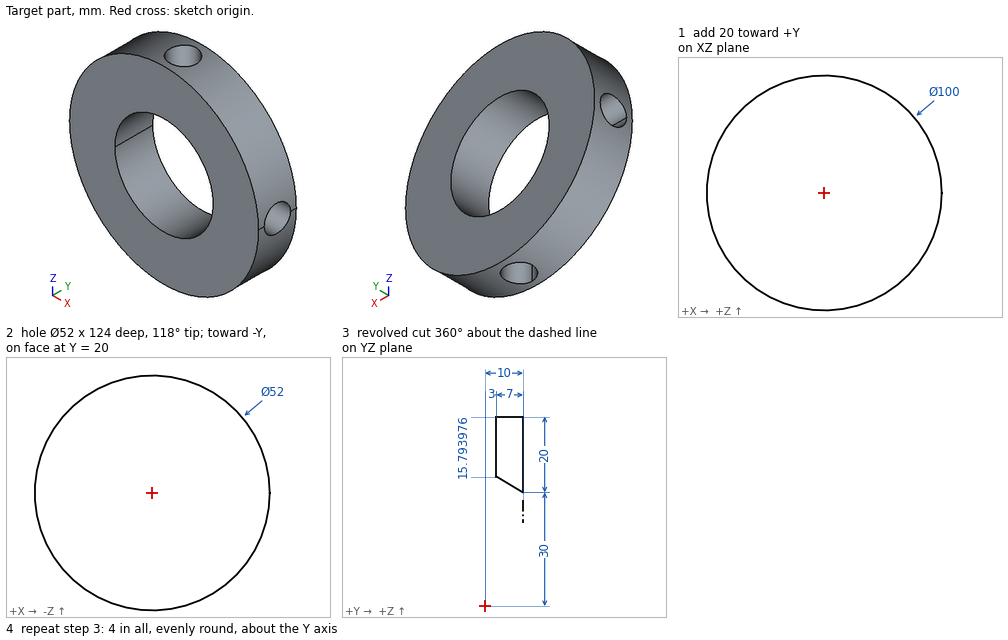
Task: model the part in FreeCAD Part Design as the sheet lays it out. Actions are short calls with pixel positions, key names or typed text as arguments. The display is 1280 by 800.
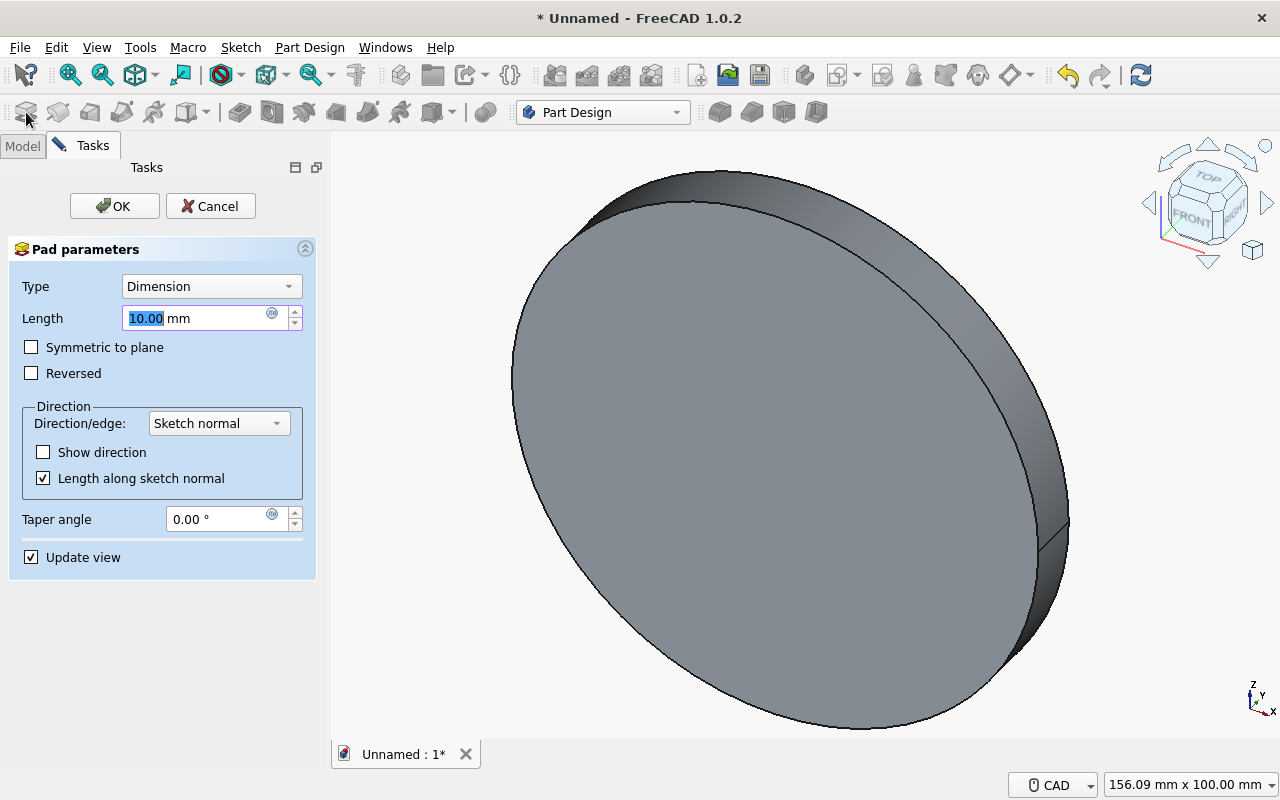
text(20)
key(Tab)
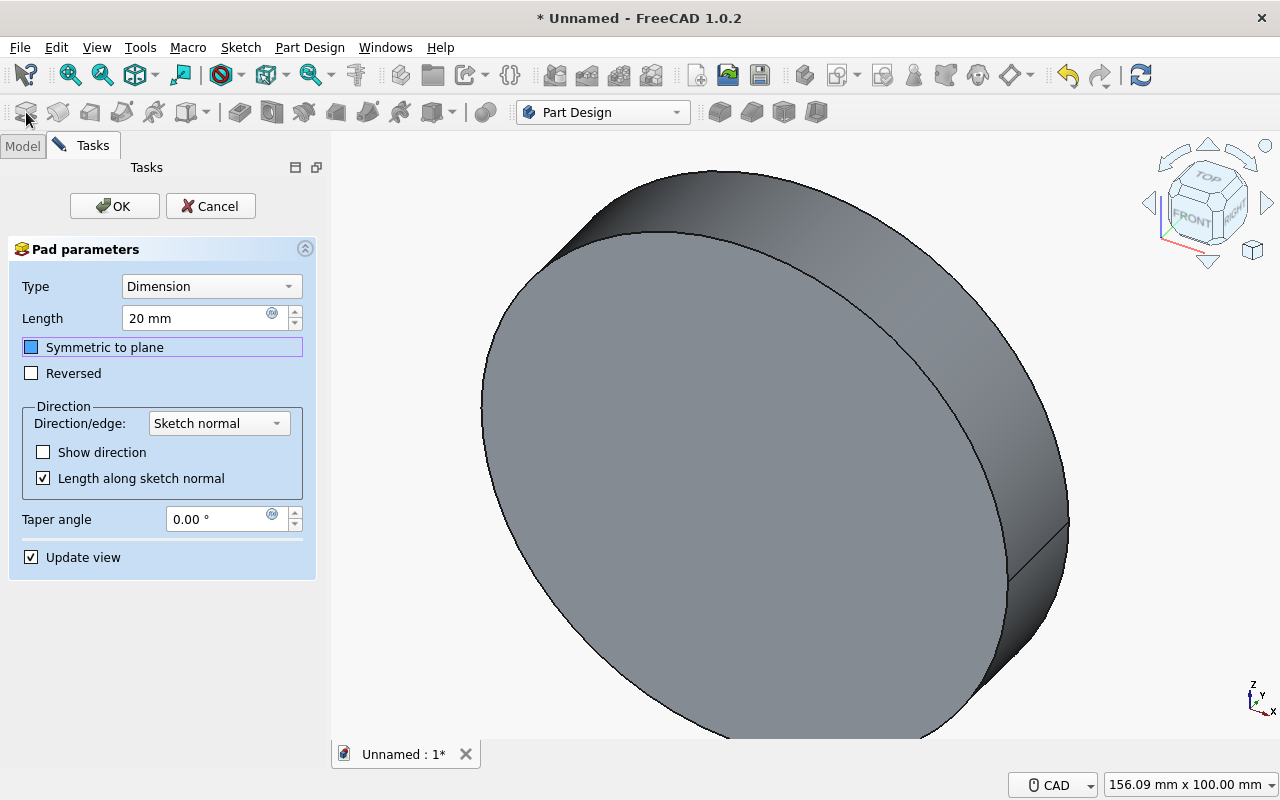
click(30, 373)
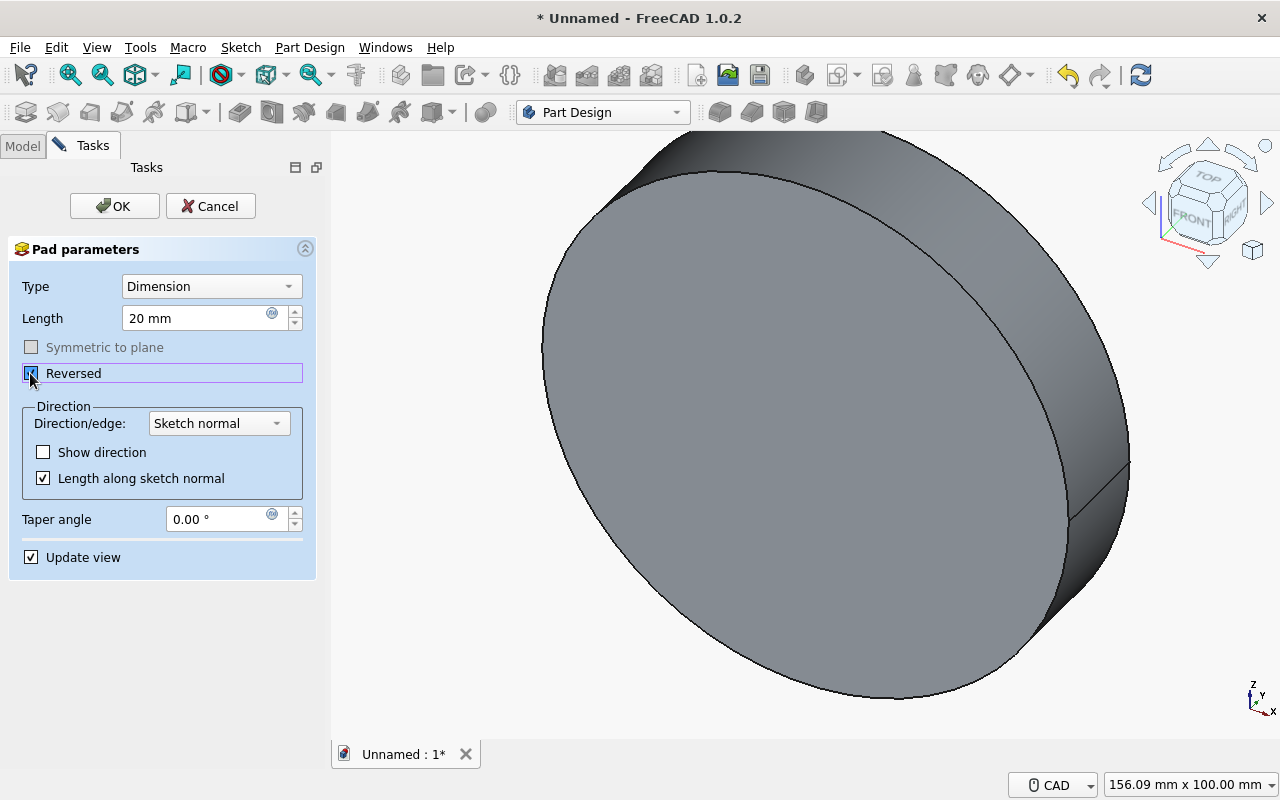
click(115, 206)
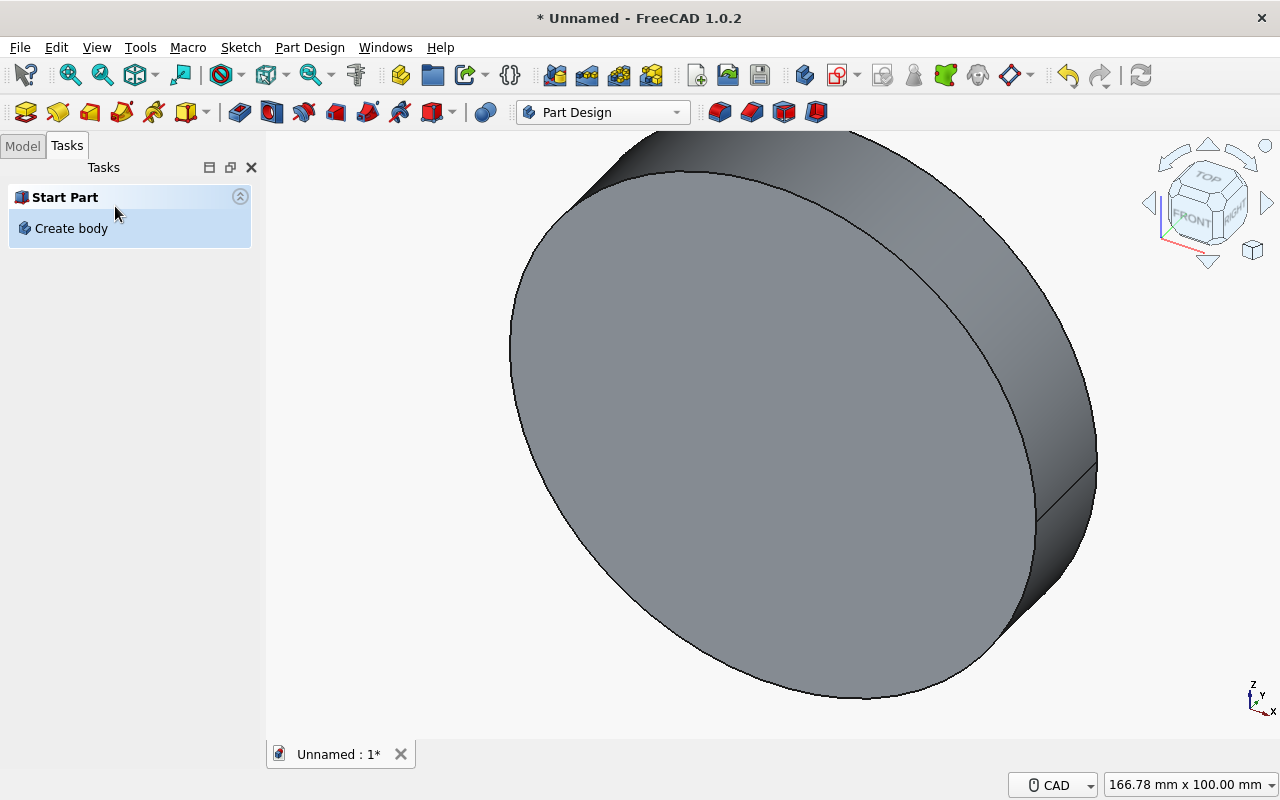
key(v)
key(f)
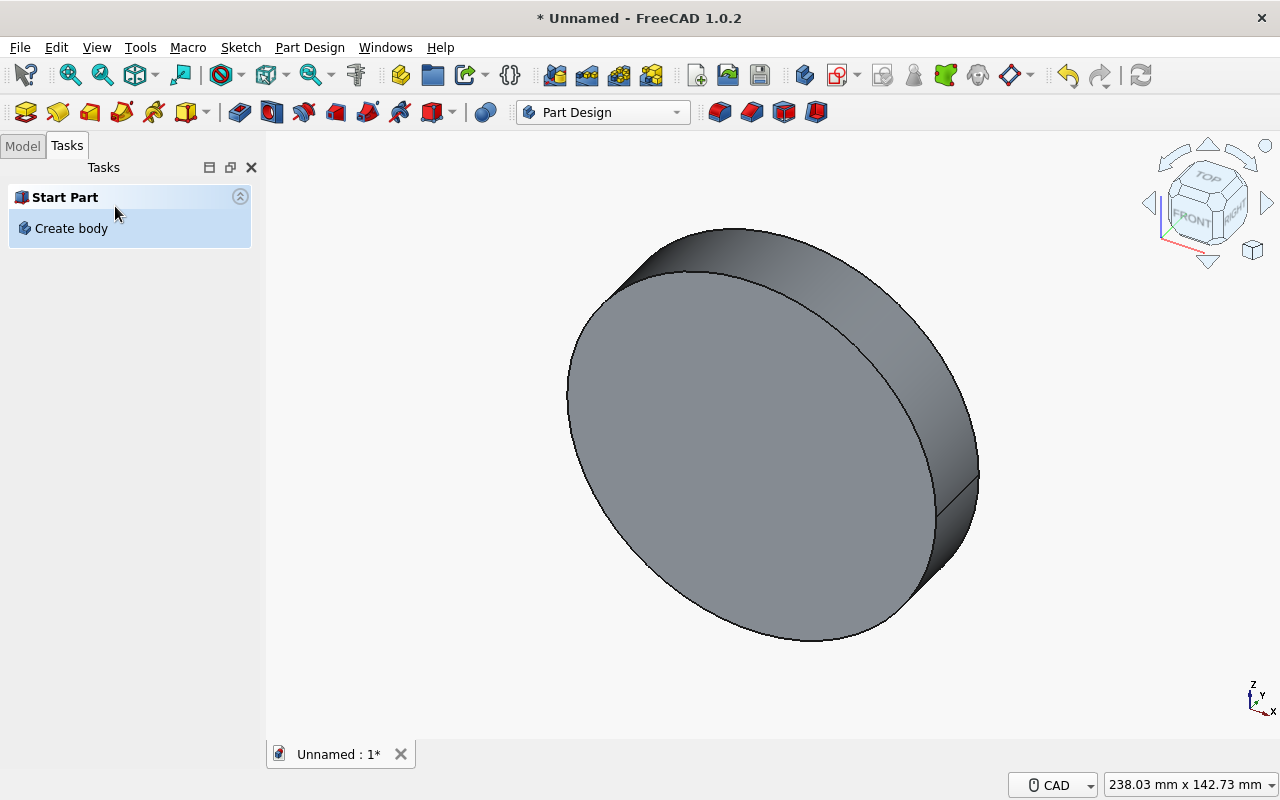
key(4)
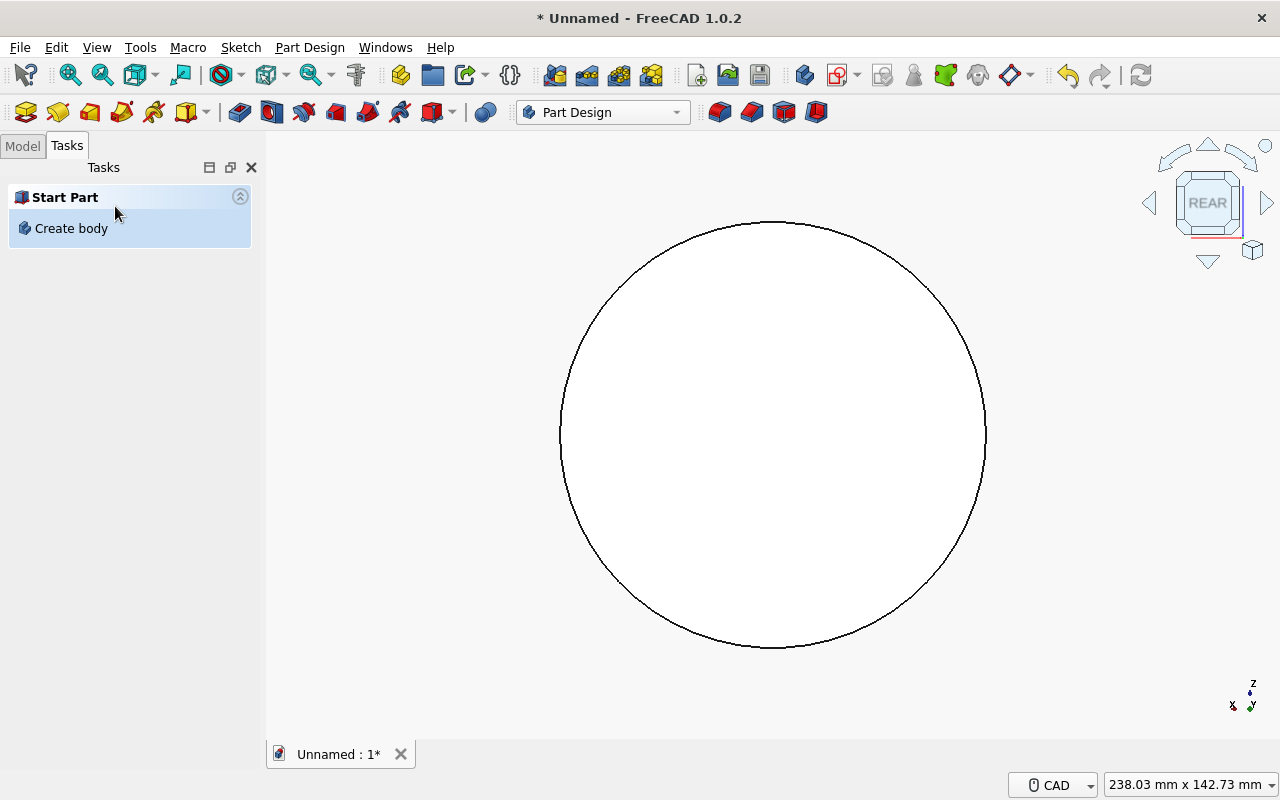
click(773, 434)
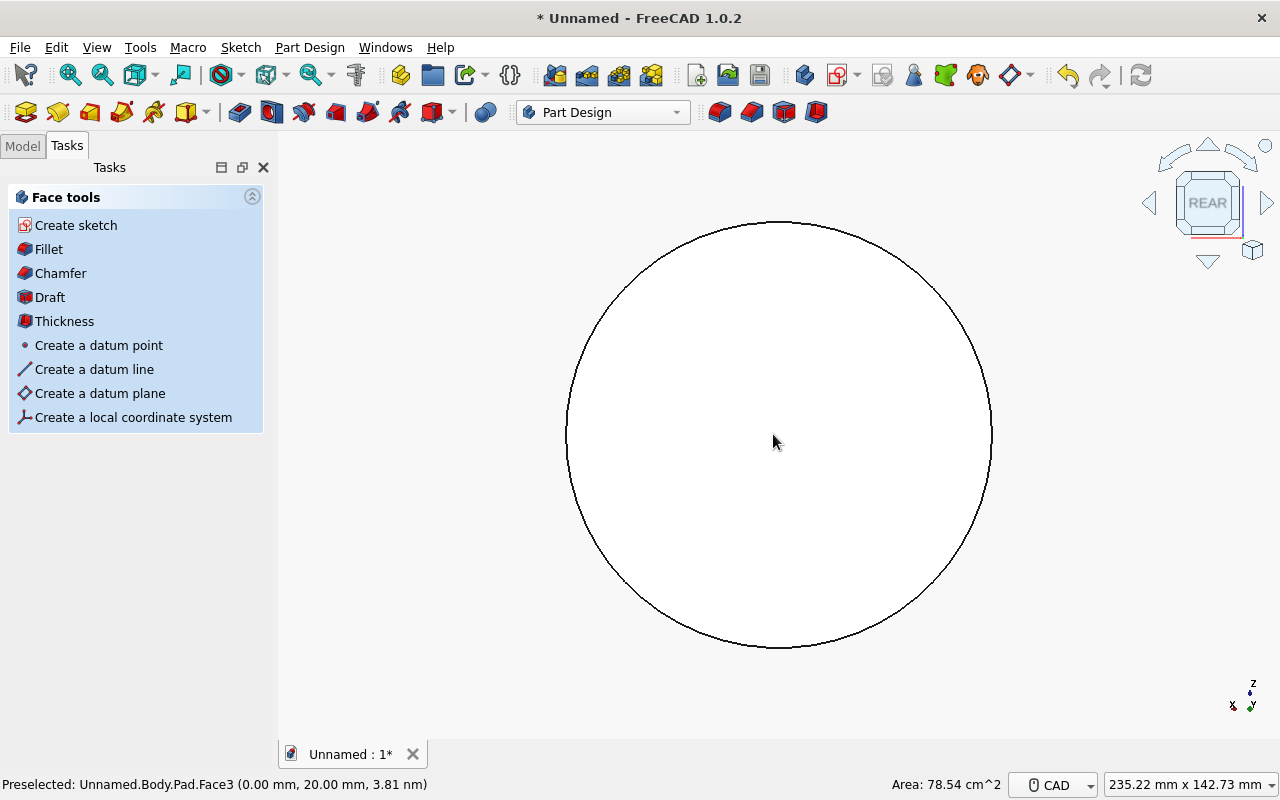
click(838, 76)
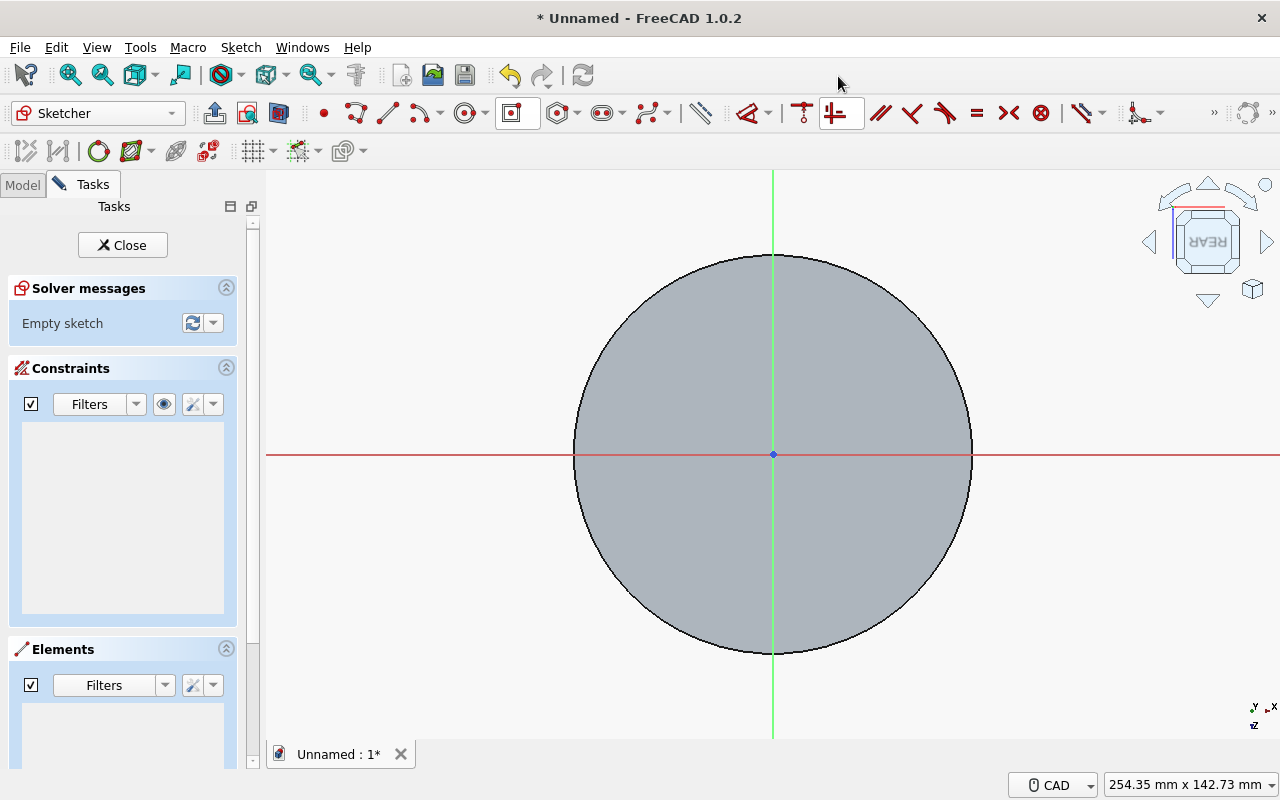
scroll(856, 455, up, 3)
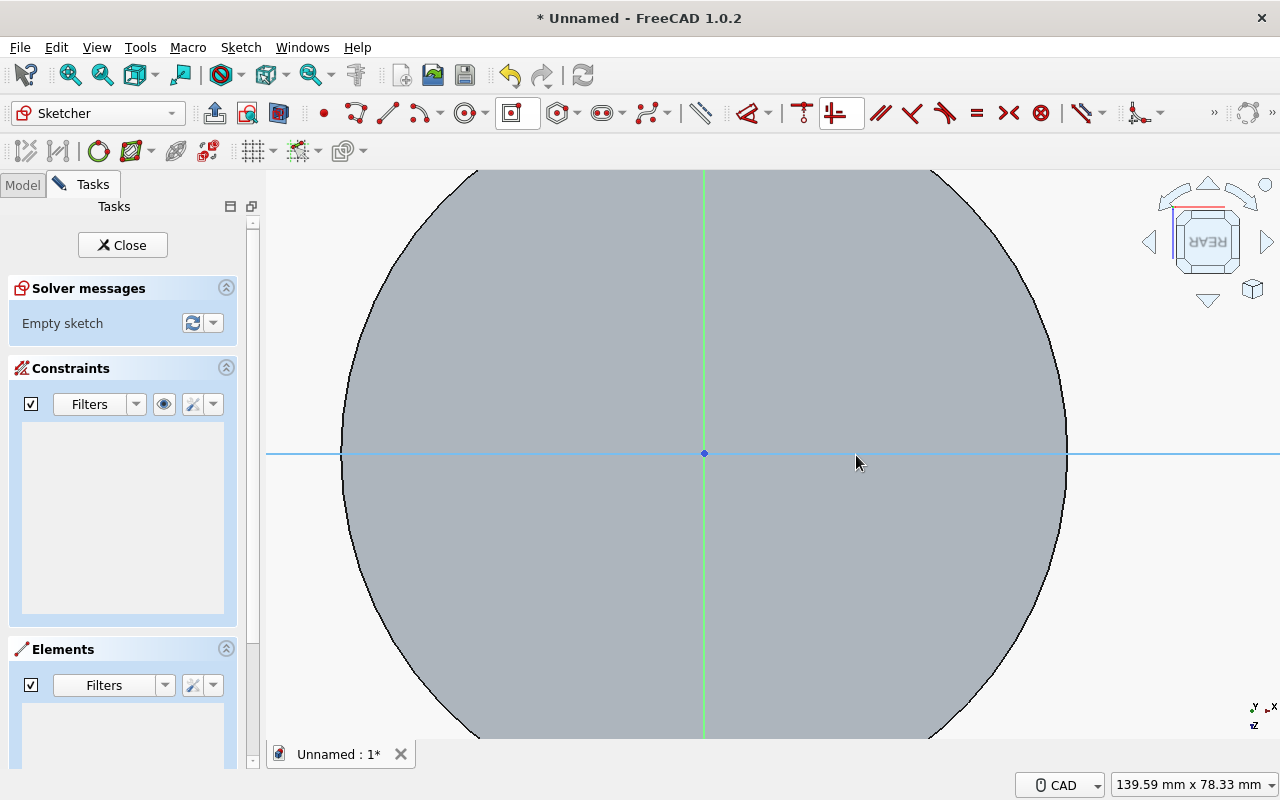
key(g)
key(c)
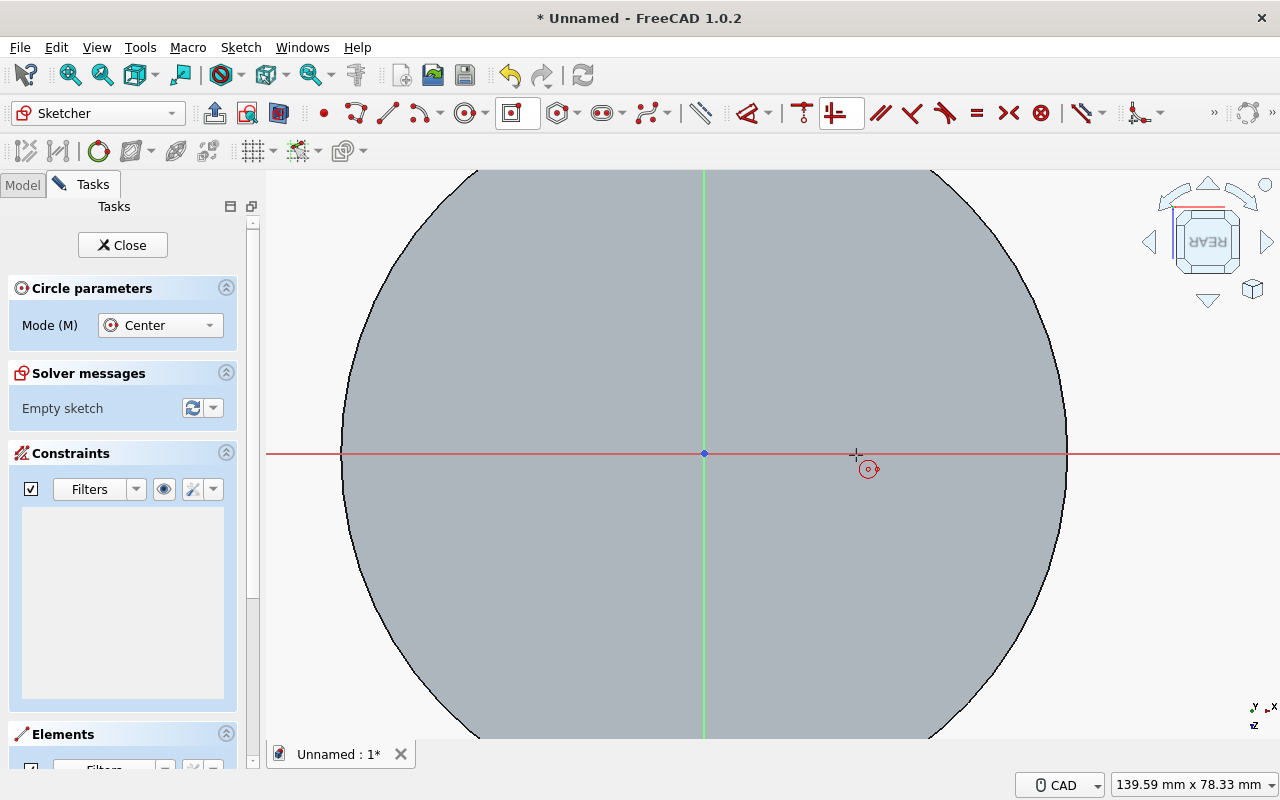
click(704, 454)
move(838, 320)